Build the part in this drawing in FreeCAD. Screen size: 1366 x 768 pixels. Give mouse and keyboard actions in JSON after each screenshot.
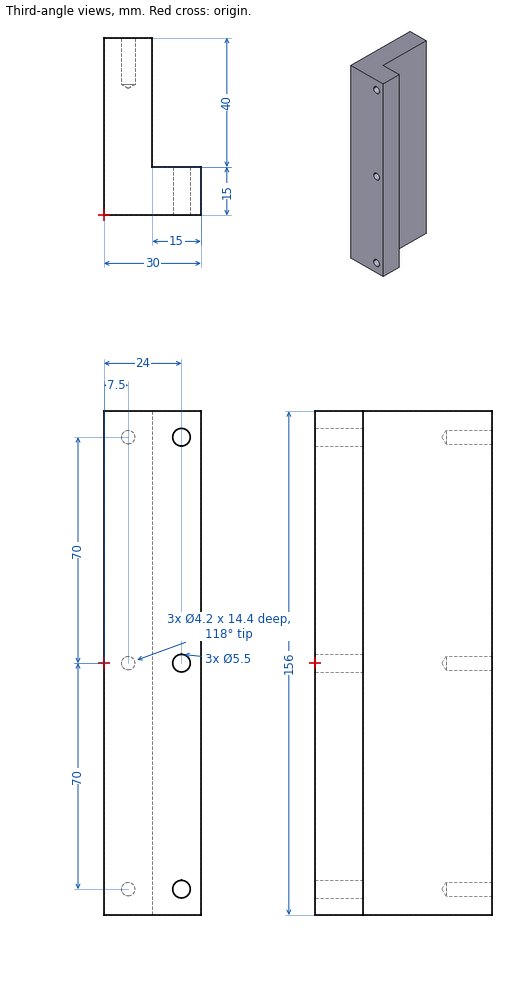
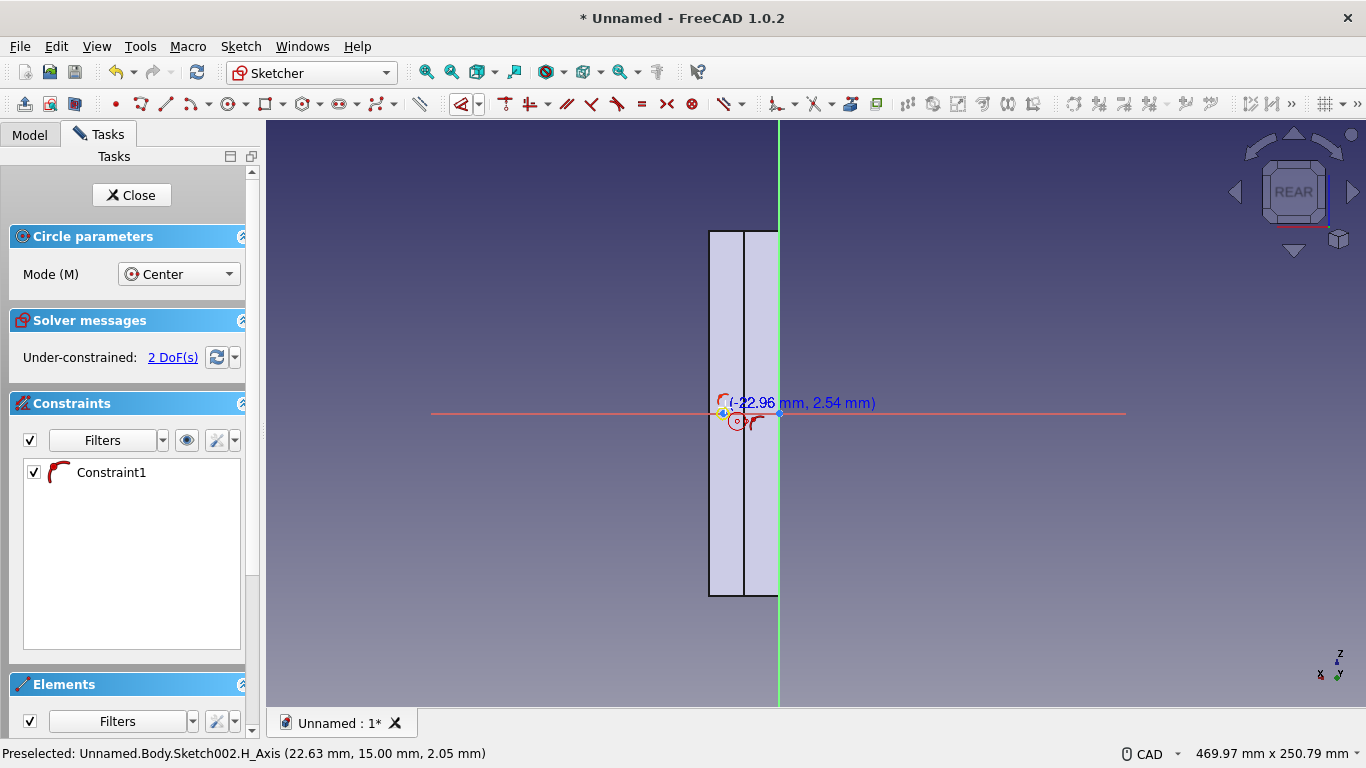
{"action": "scroll", "coordinate": [723, 577], "scroll_direction": "up", "scroll_amount": 7}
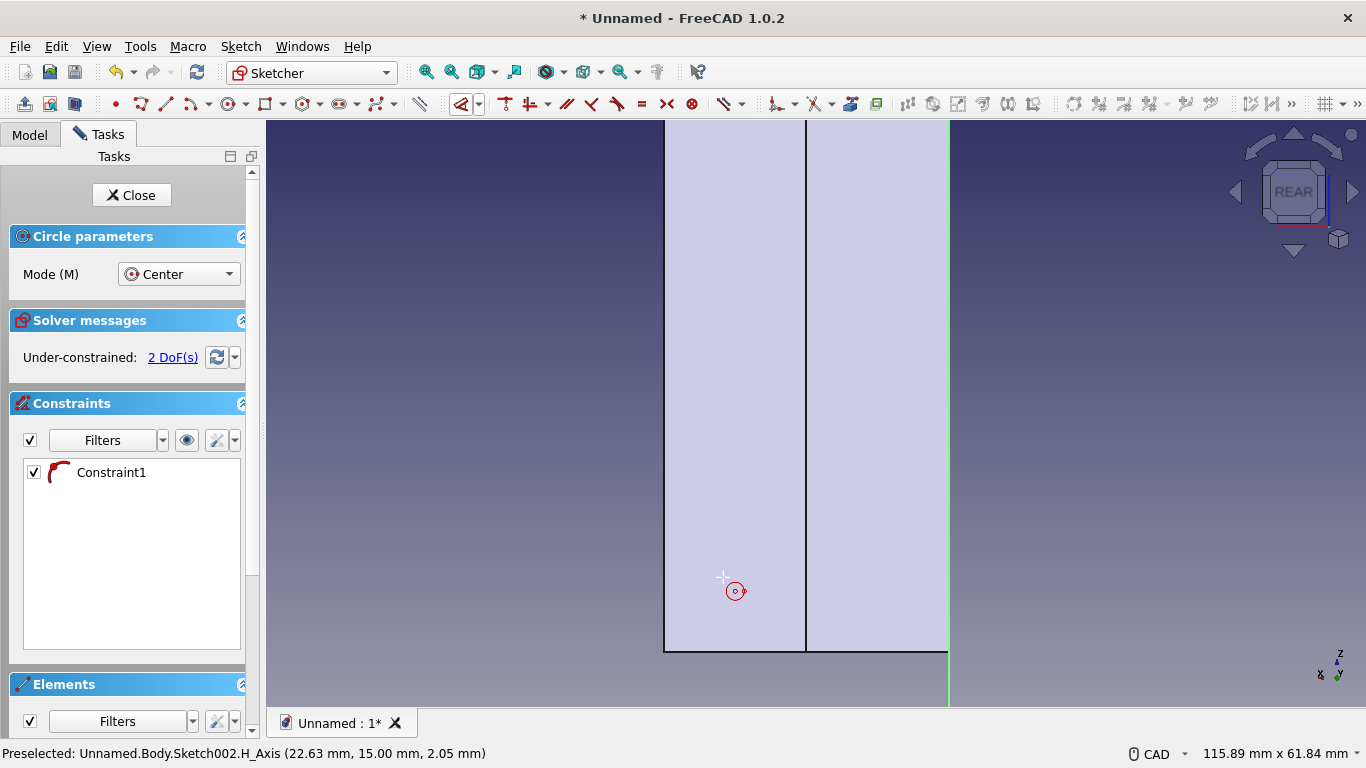
{"action": "scroll", "coordinate": [723, 578], "scroll_direction": "down", "scroll_amount": 7}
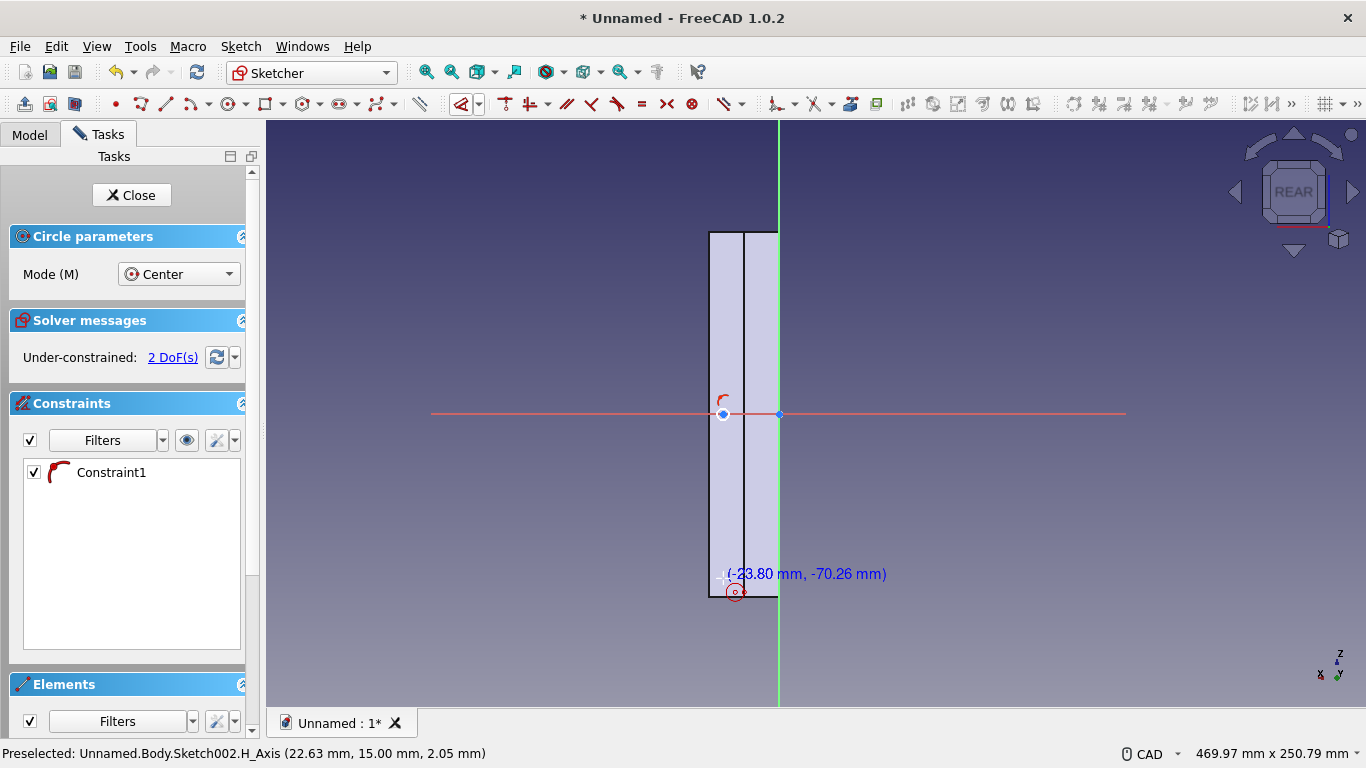
{"action": "left_click", "coordinate": [723, 578]}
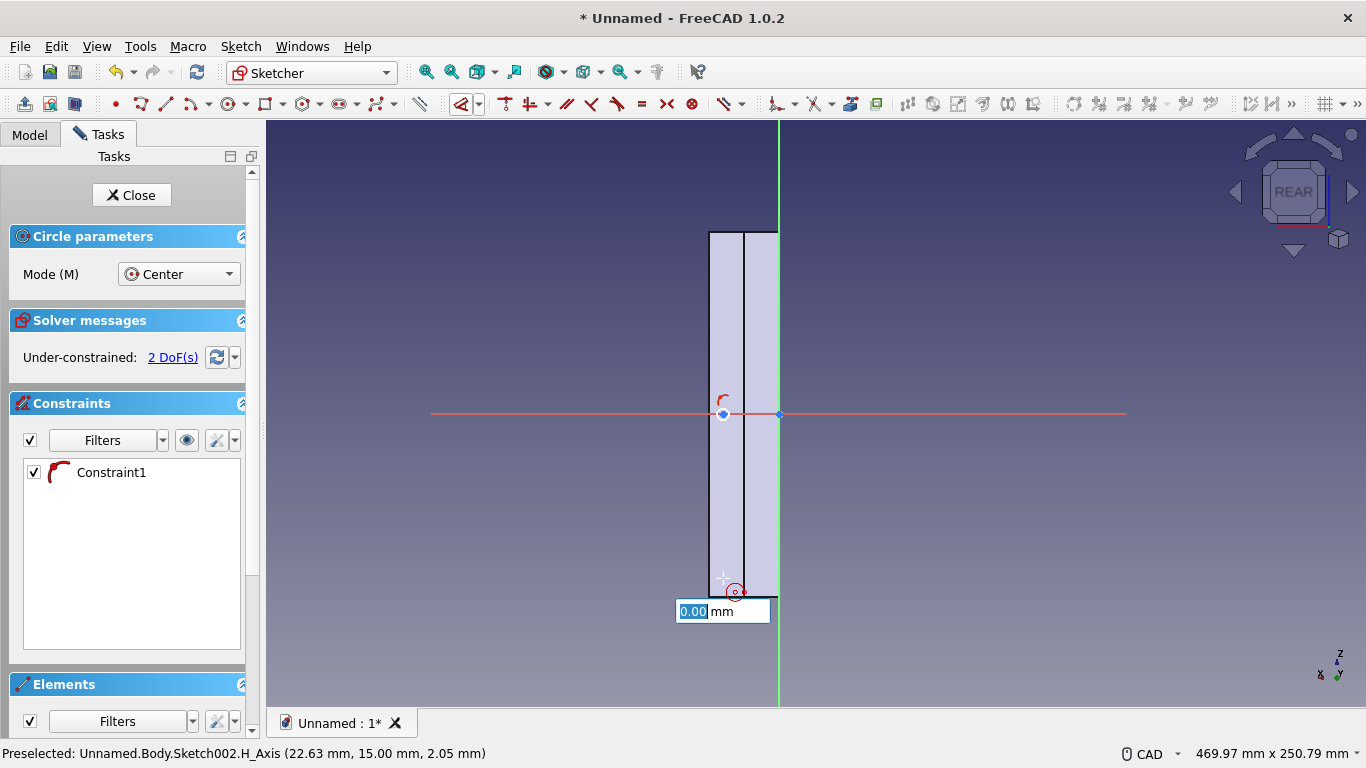
{"action": "scroll", "coordinate": [727, 574], "scroll_direction": "up", "scroll_amount": 5}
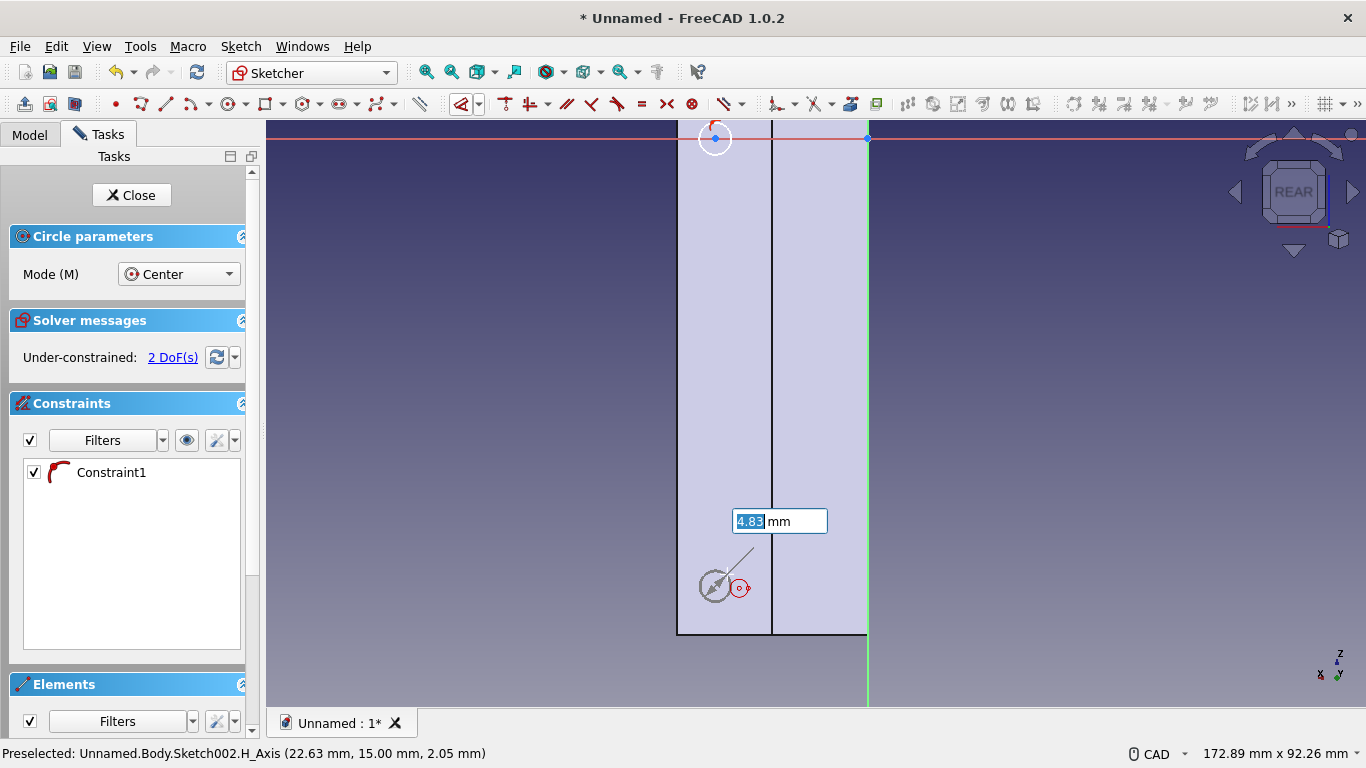
{"action": "left_click", "coordinate": [727, 572]}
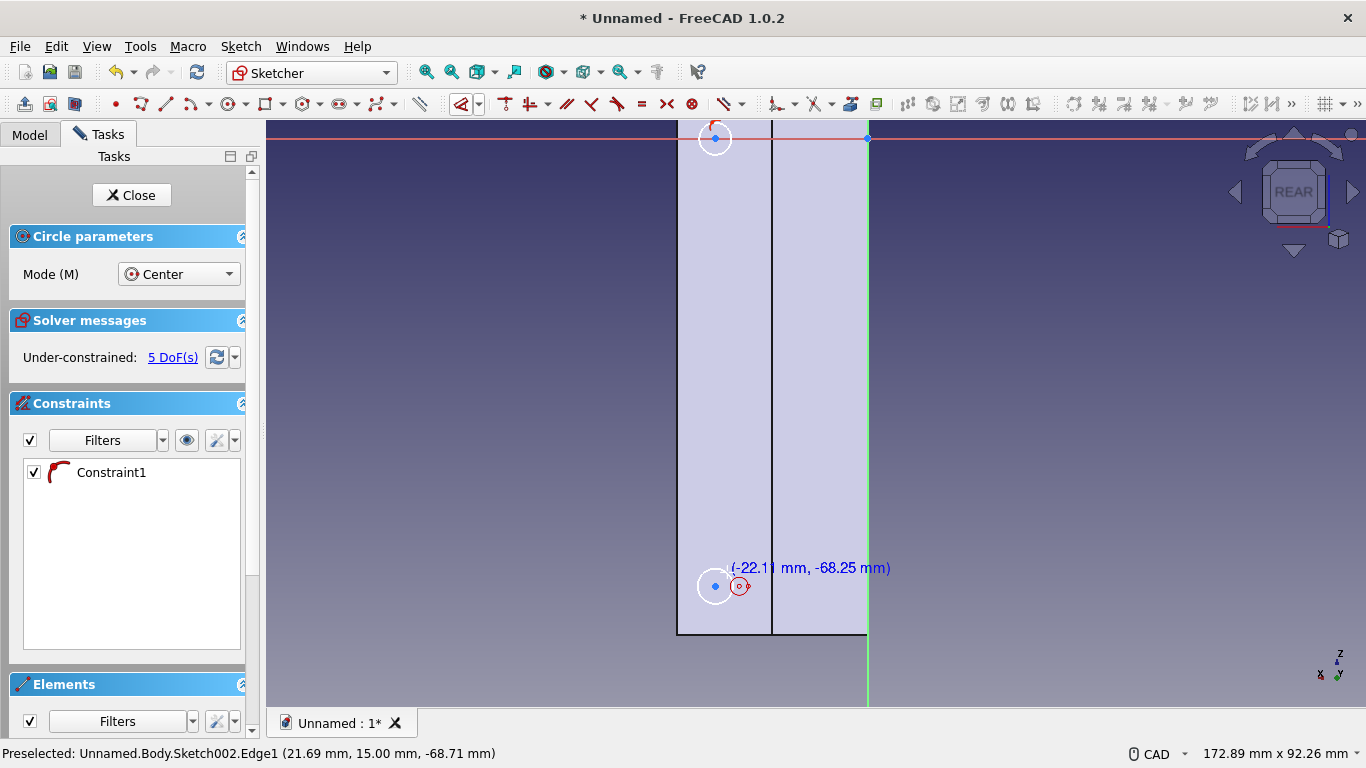
{"action": "scroll", "coordinate": [727, 573], "scroll_direction": "down", "scroll_amount": 5}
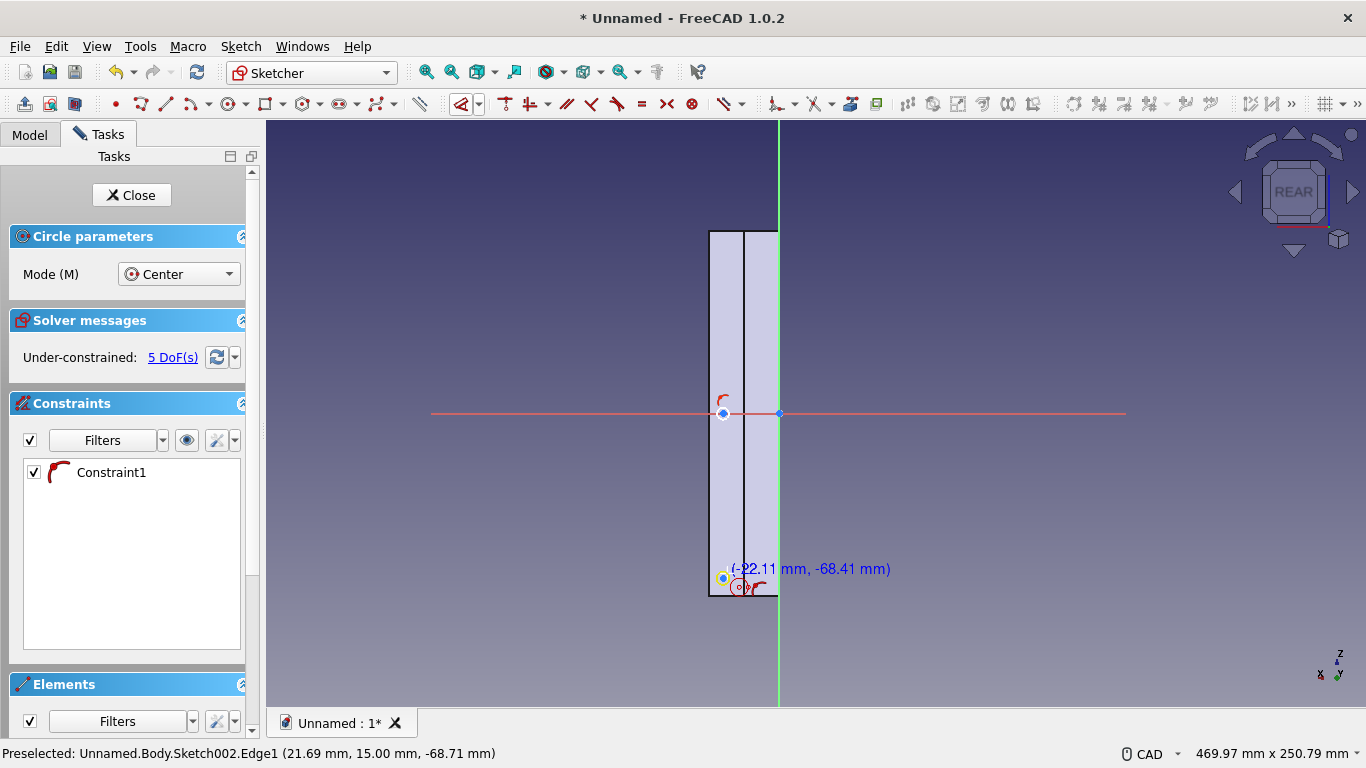
{"action": "scroll", "coordinate": [723, 250], "scroll_direction": "up", "scroll_amount": 7}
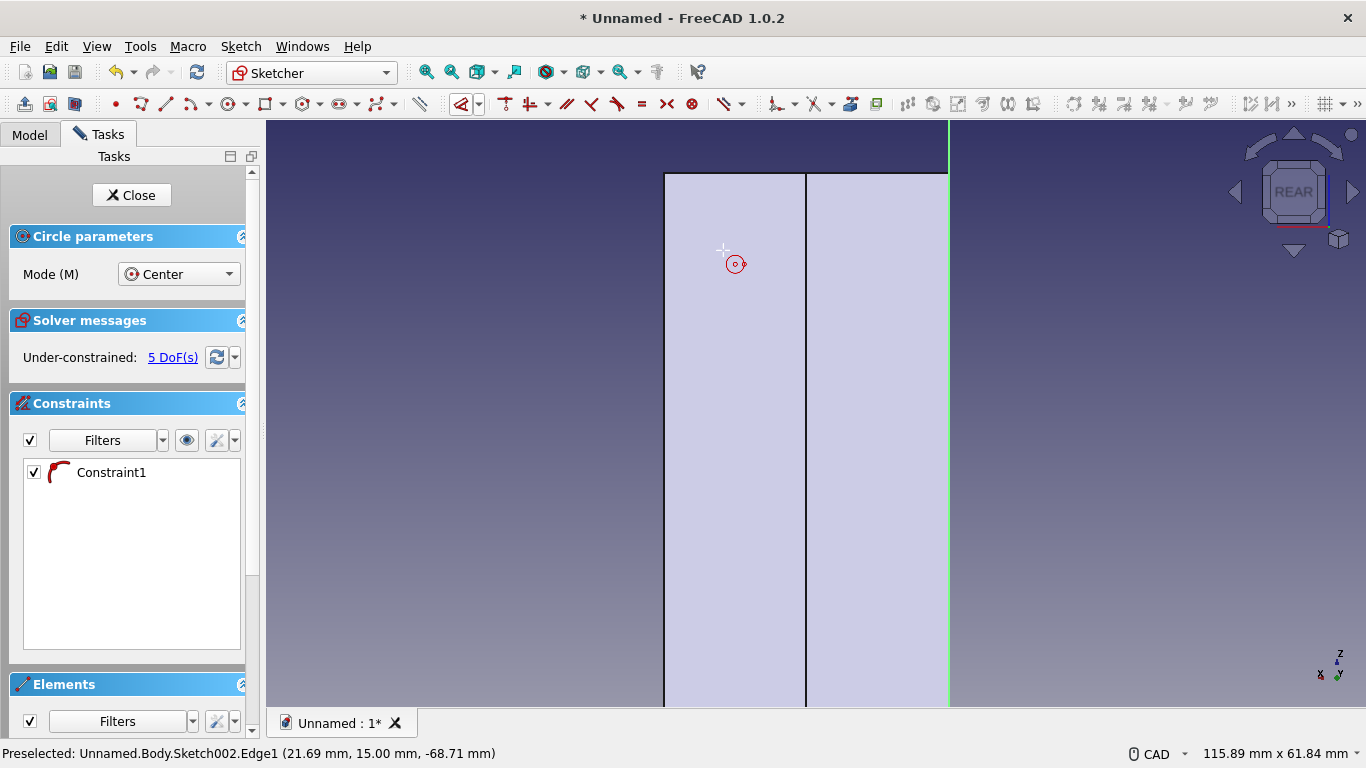
{"action": "scroll", "coordinate": [723, 250], "scroll_direction": "down", "scroll_amount": 7}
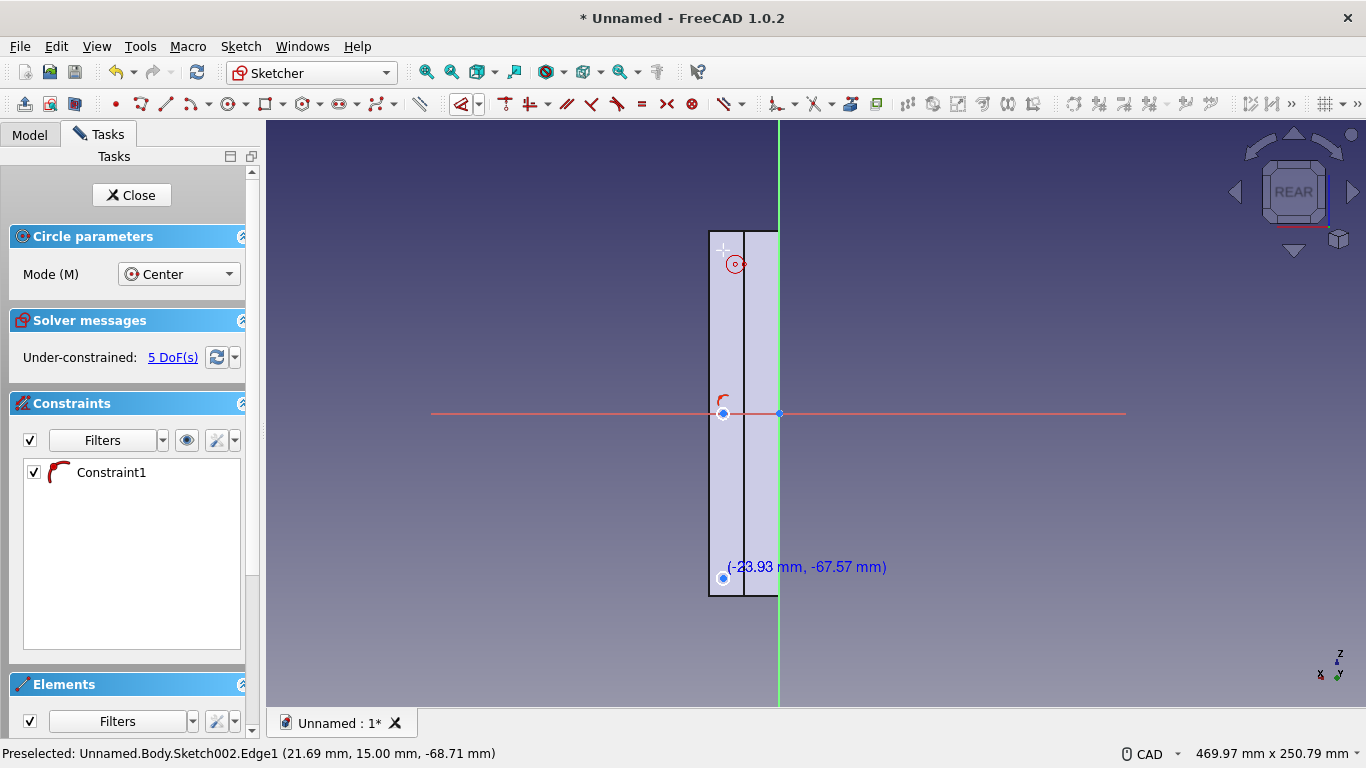
{"action": "left_click", "coordinate": [723, 250]}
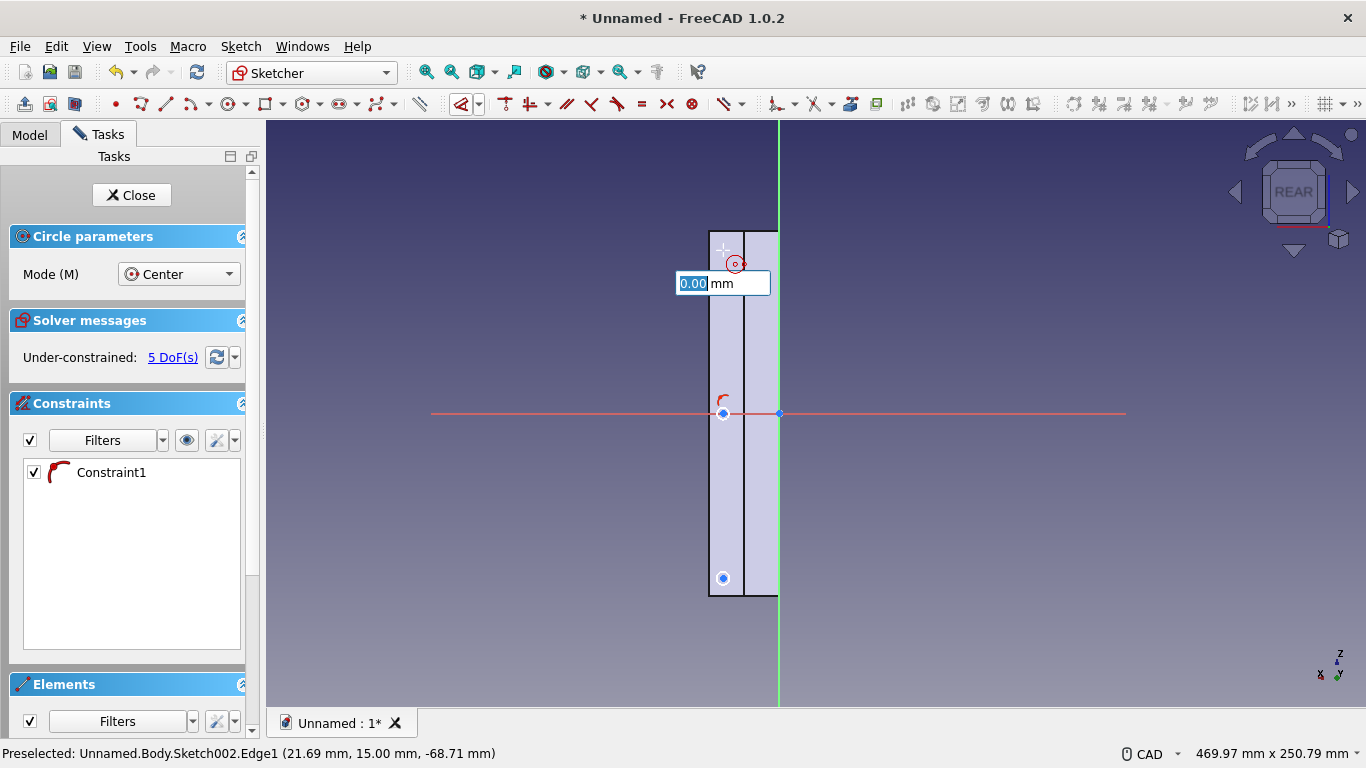
{"action": "scroll", "coordinate": [727, 245], "scroll_direction": "up", "scroll_amount": 5}